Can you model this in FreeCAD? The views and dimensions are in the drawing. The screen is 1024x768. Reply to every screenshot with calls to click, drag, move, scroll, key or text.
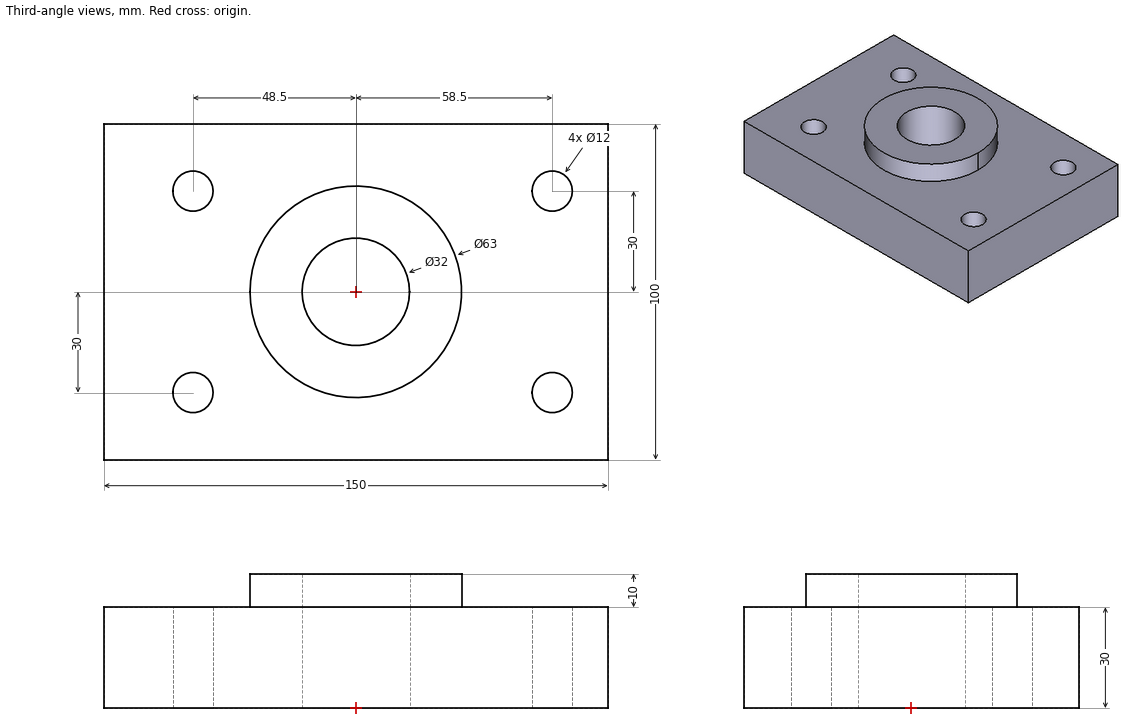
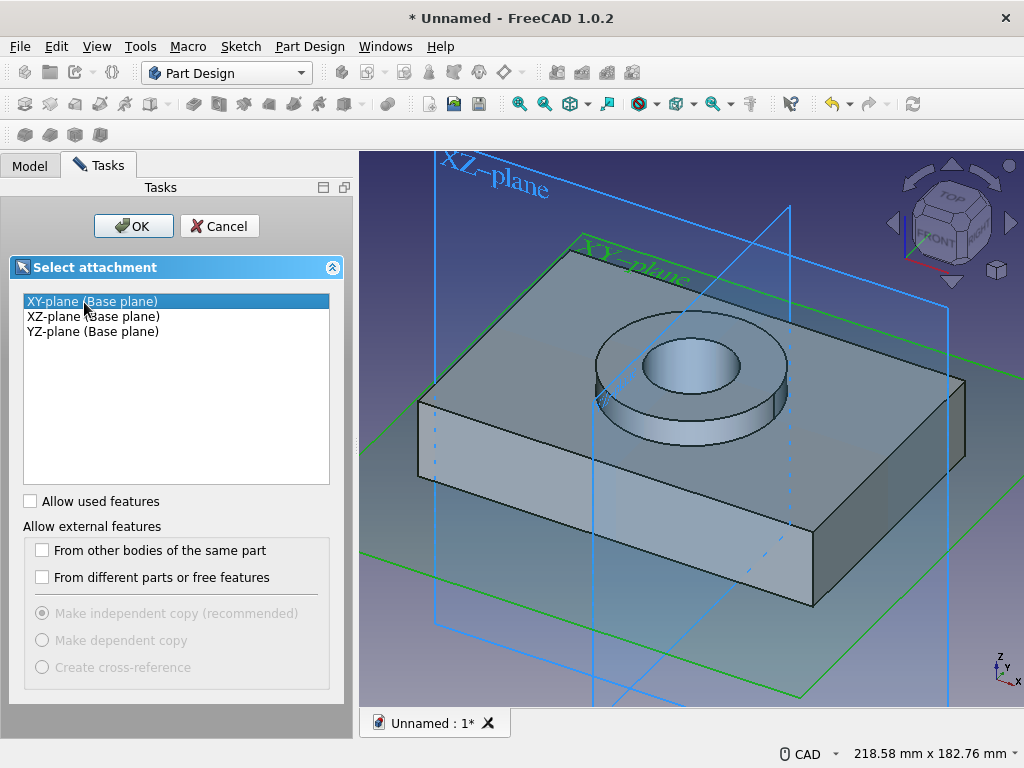
click(134, 226)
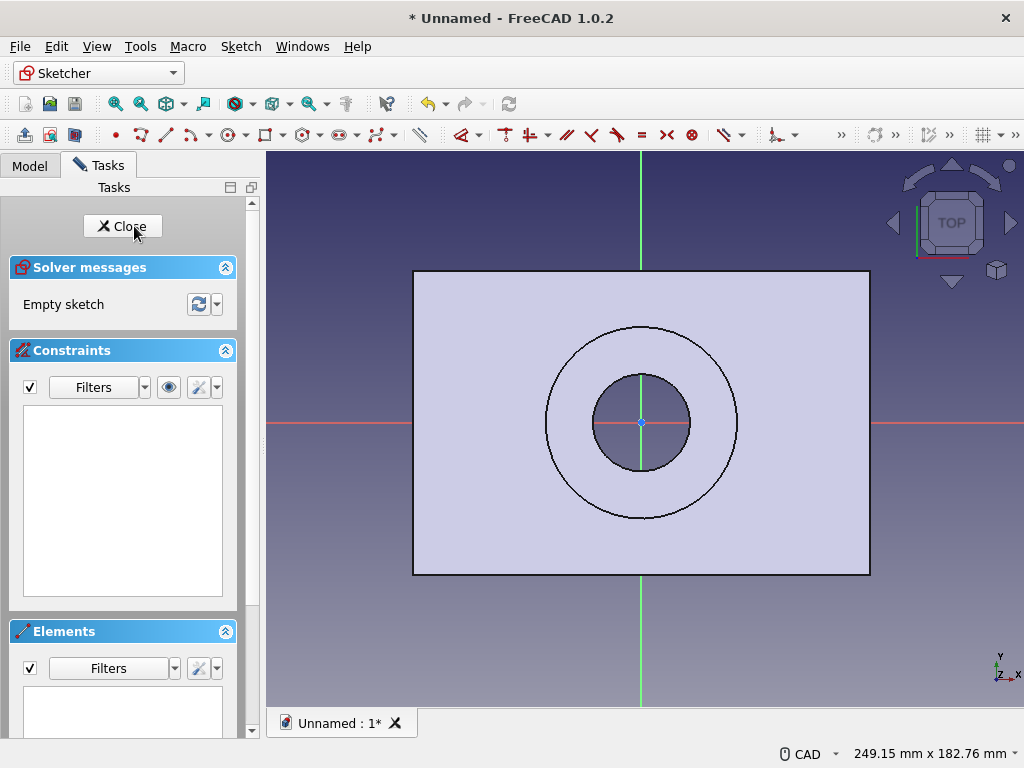
click(75, 136)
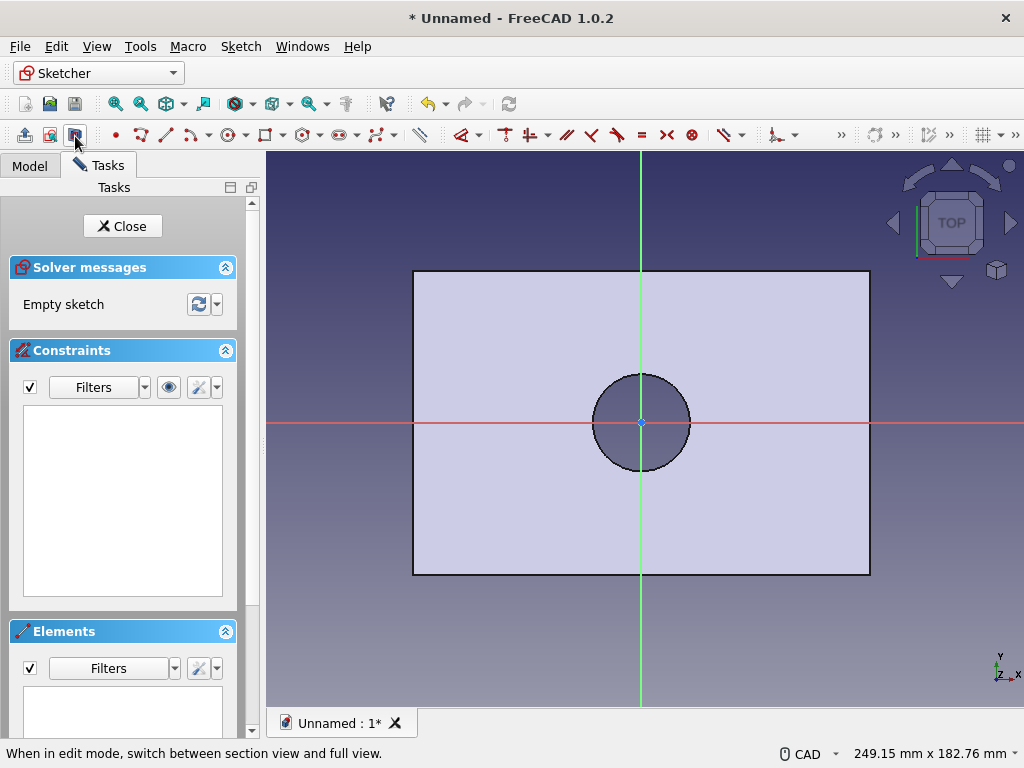
scroll(294, 457, down, 1)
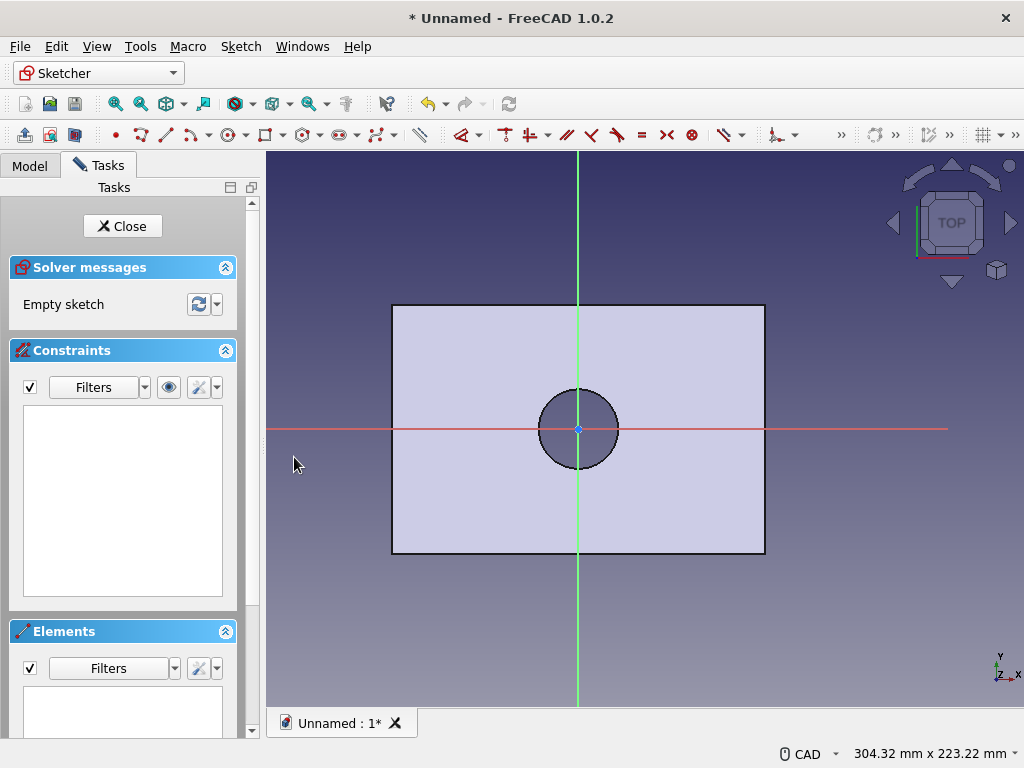
click(228, 136)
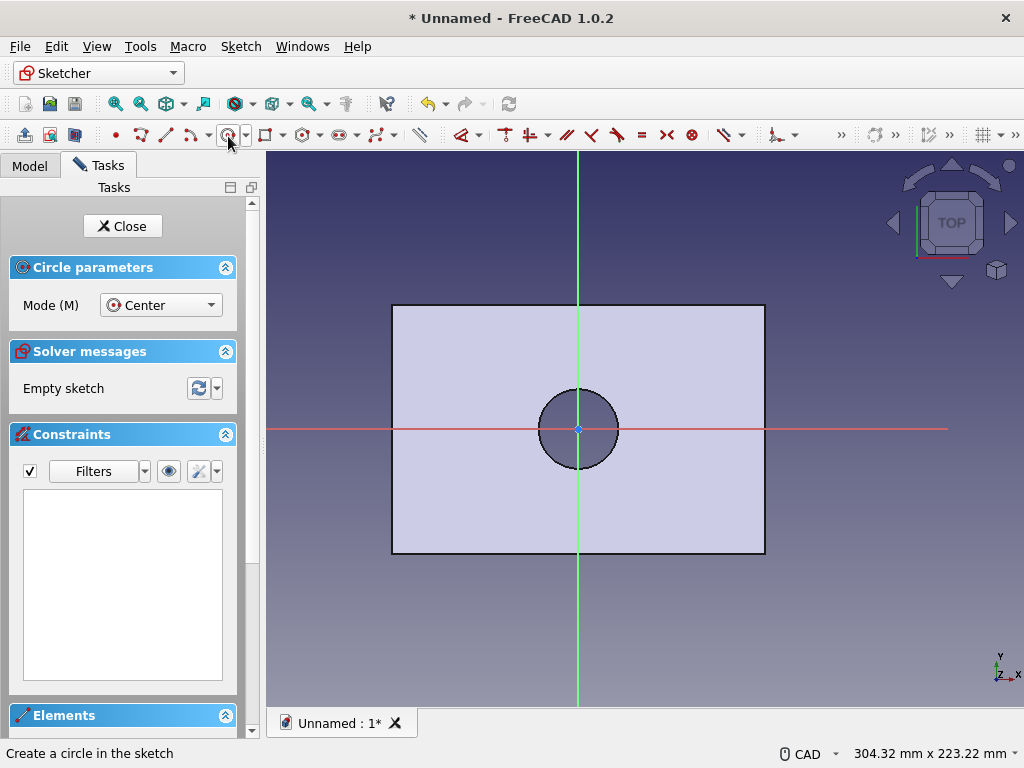
scroll(724, 354, up, 3)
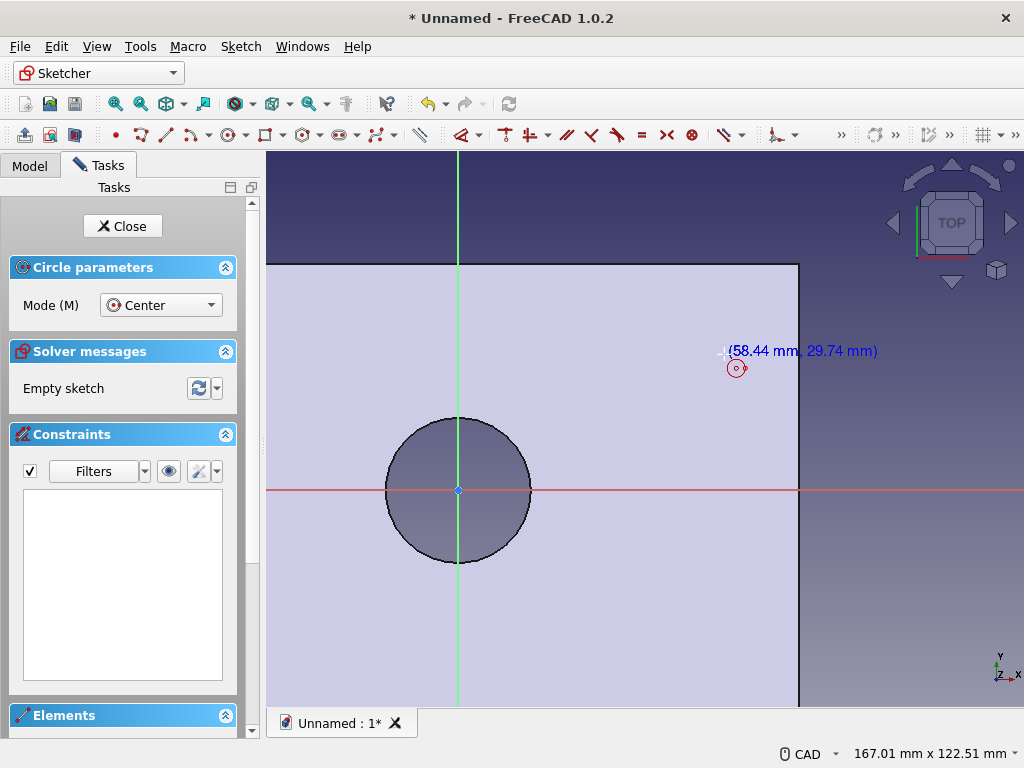
click(724, 354)
move(743, 335)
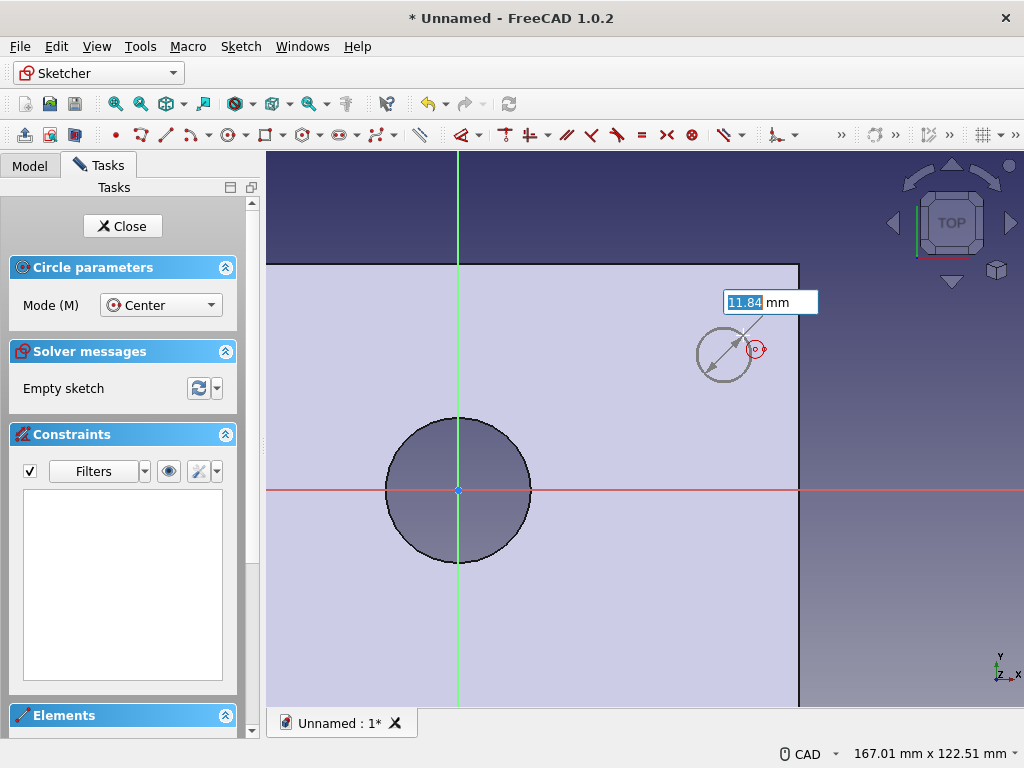
text(12)
key(Return)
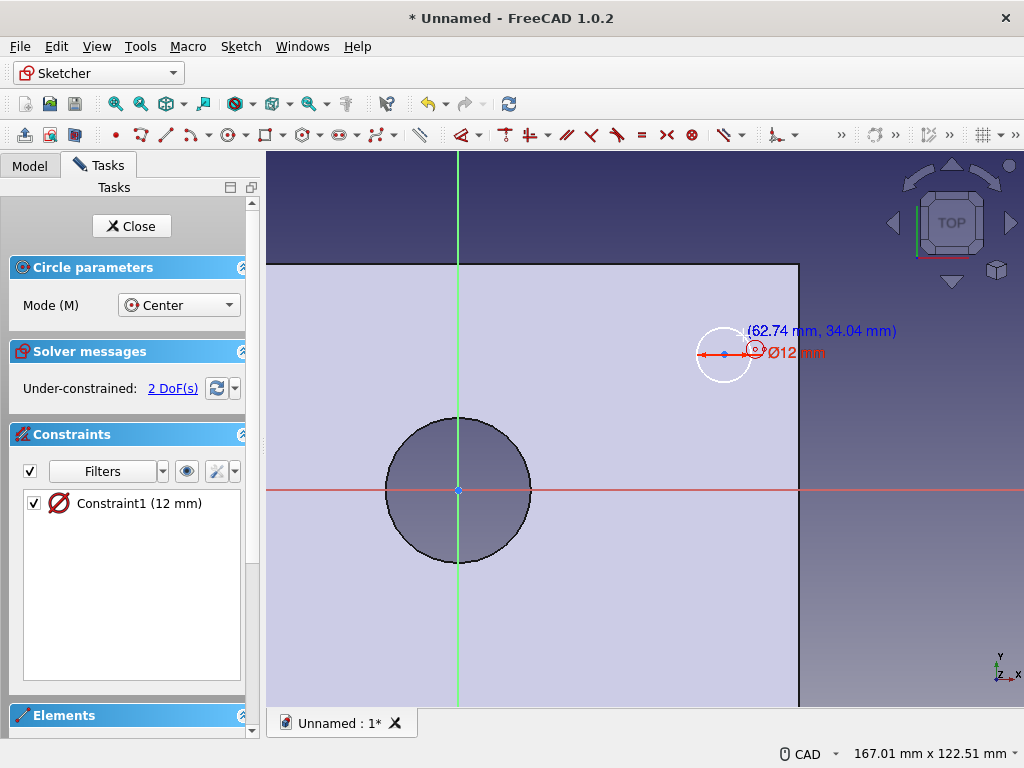
scroll(771, 304, down, 2)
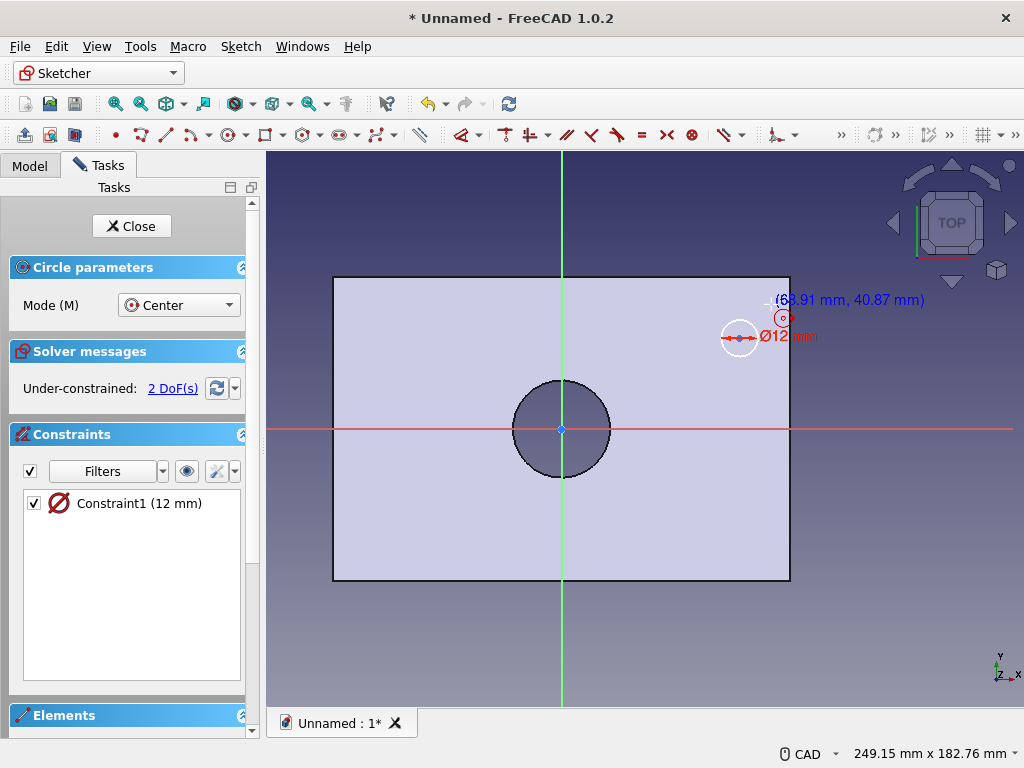
scroll(414, 338, up, 2)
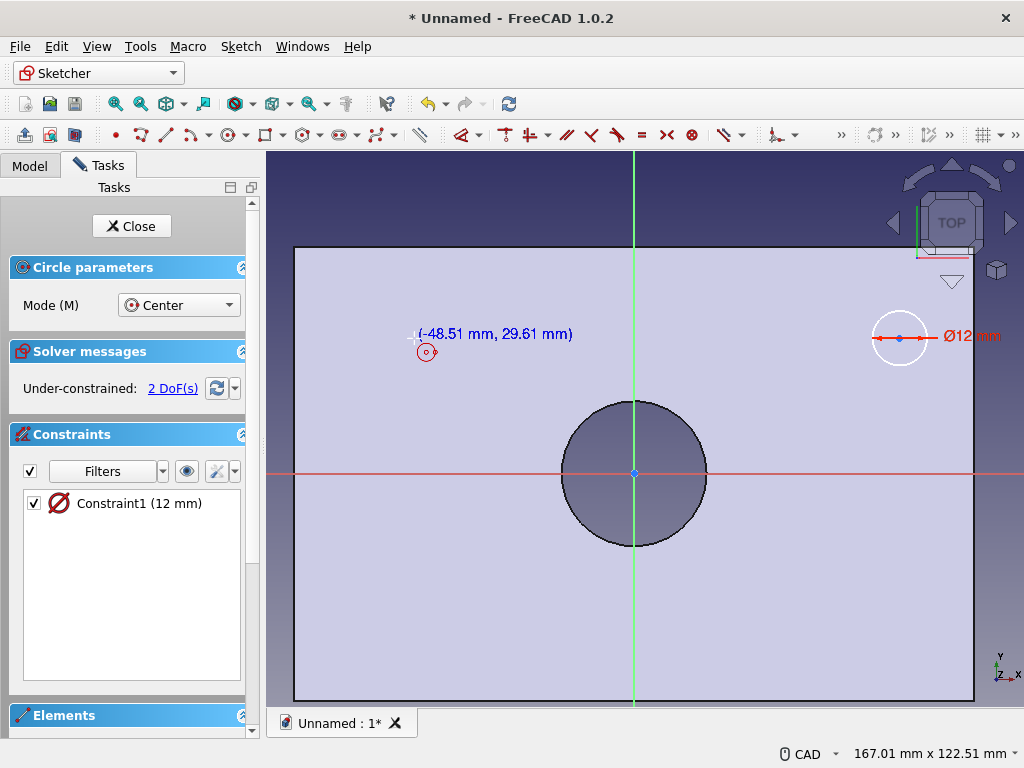
click(414, 338)
move(433, 318)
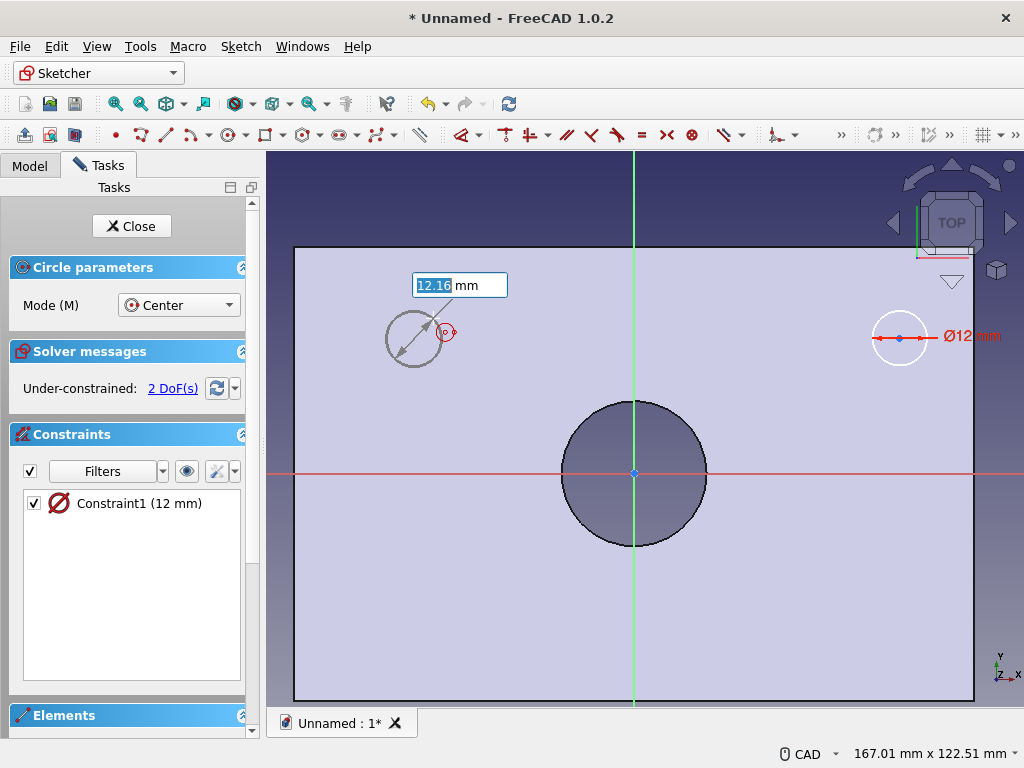
text(12)
key(Return)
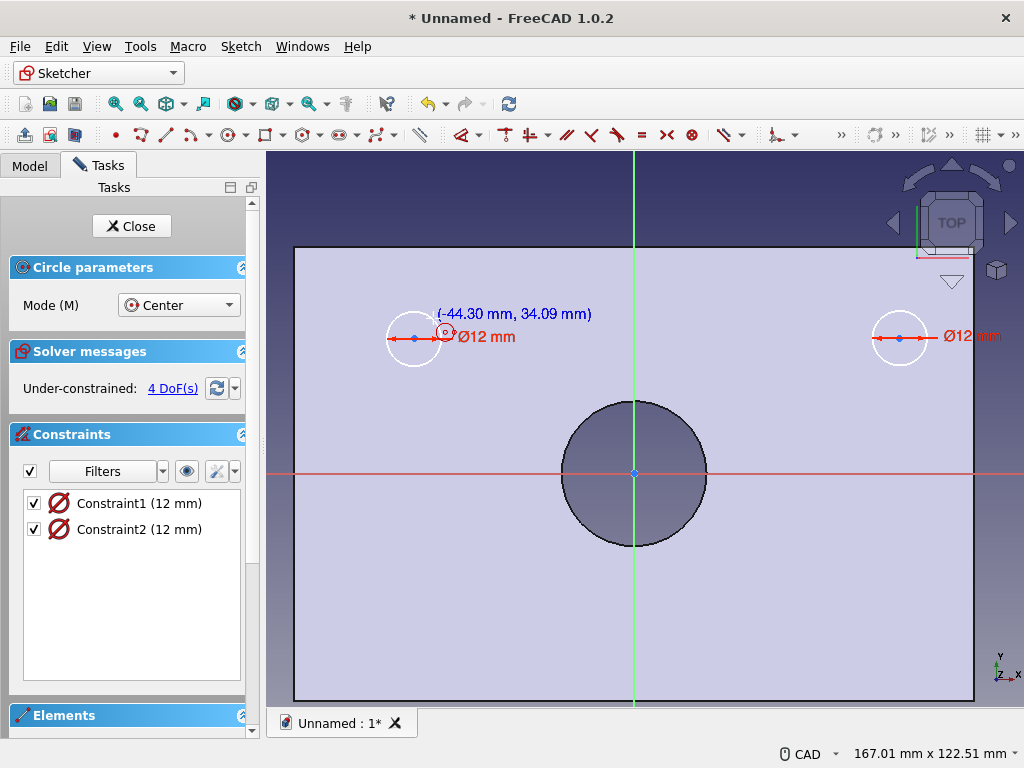
click(414, 610)
move(433, 591)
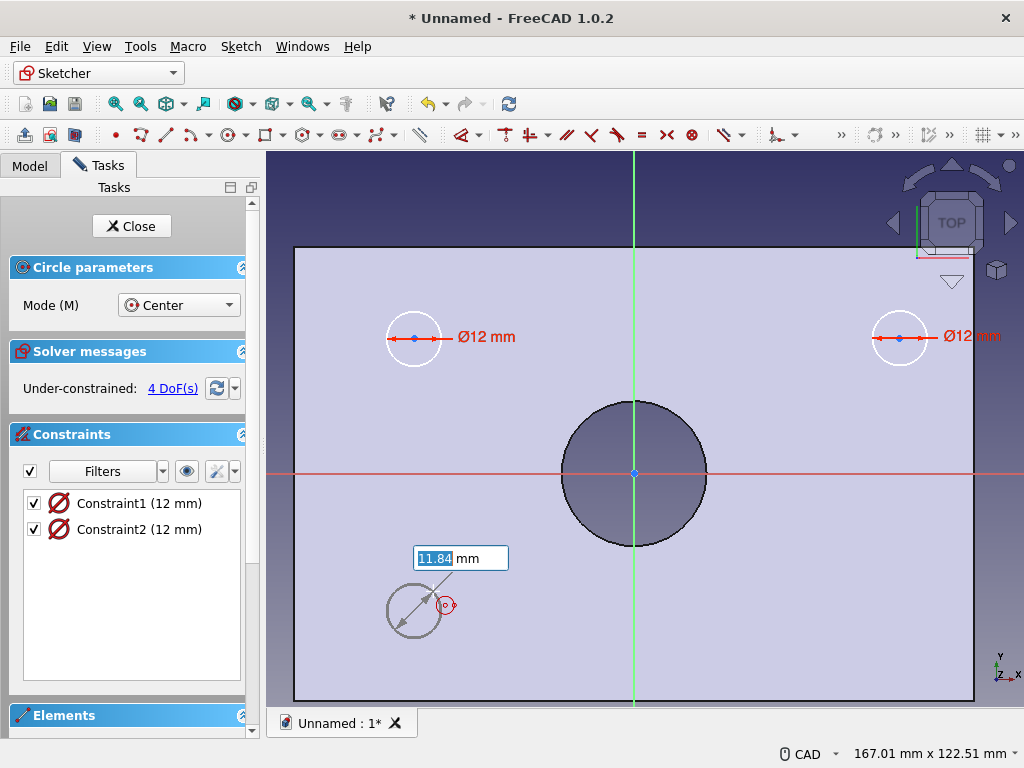
text(12)
key(Return)